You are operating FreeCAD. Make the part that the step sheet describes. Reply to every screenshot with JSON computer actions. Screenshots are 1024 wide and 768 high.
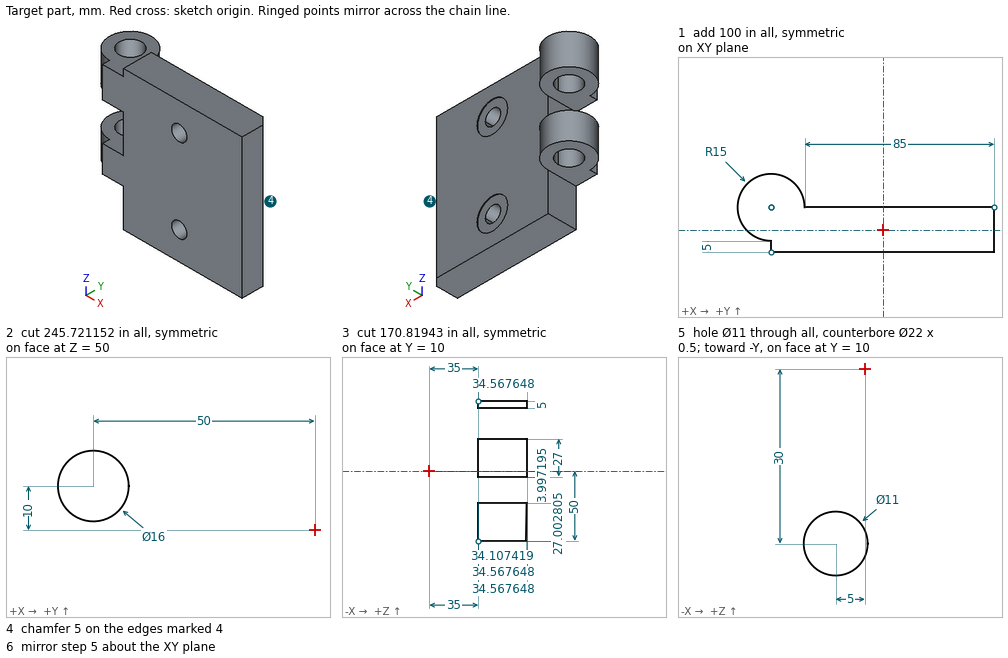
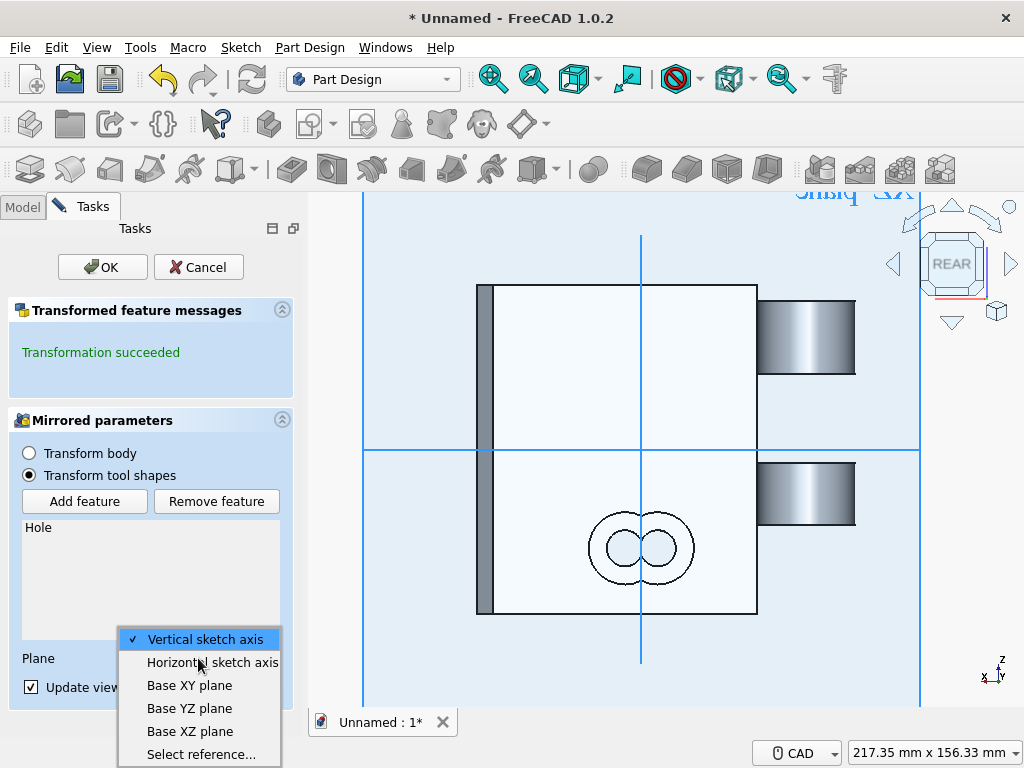
{"action": "left_click", "coordinate": [198, 686]}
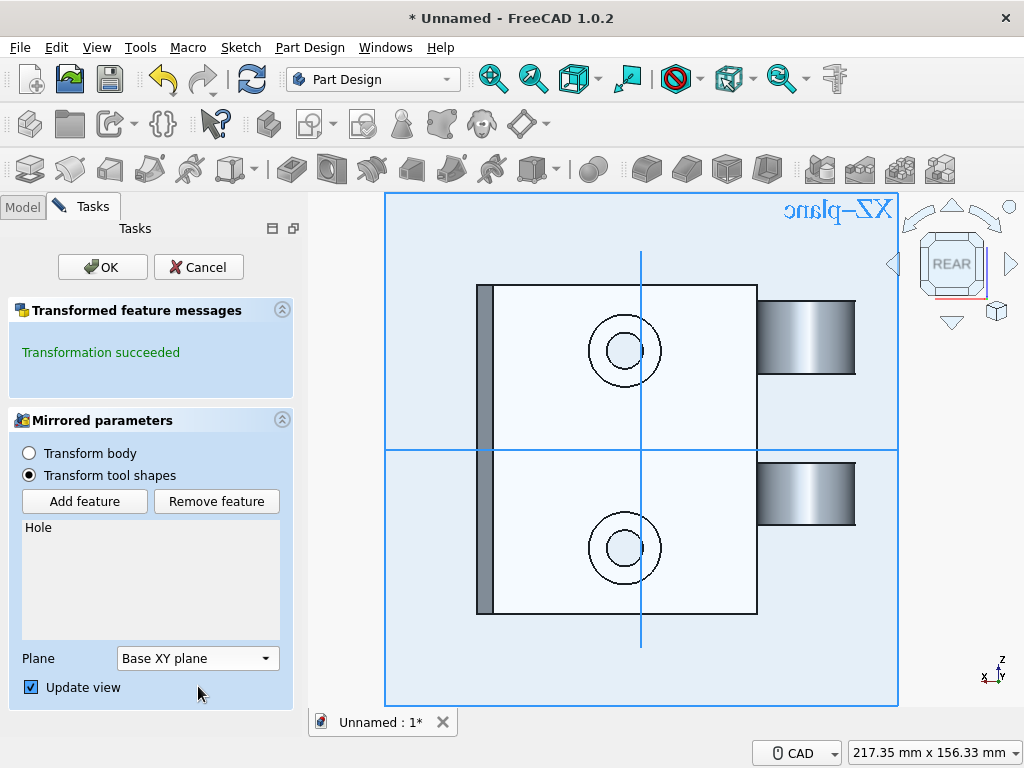
{"action": "left_click", "coordinate": [103, 267]}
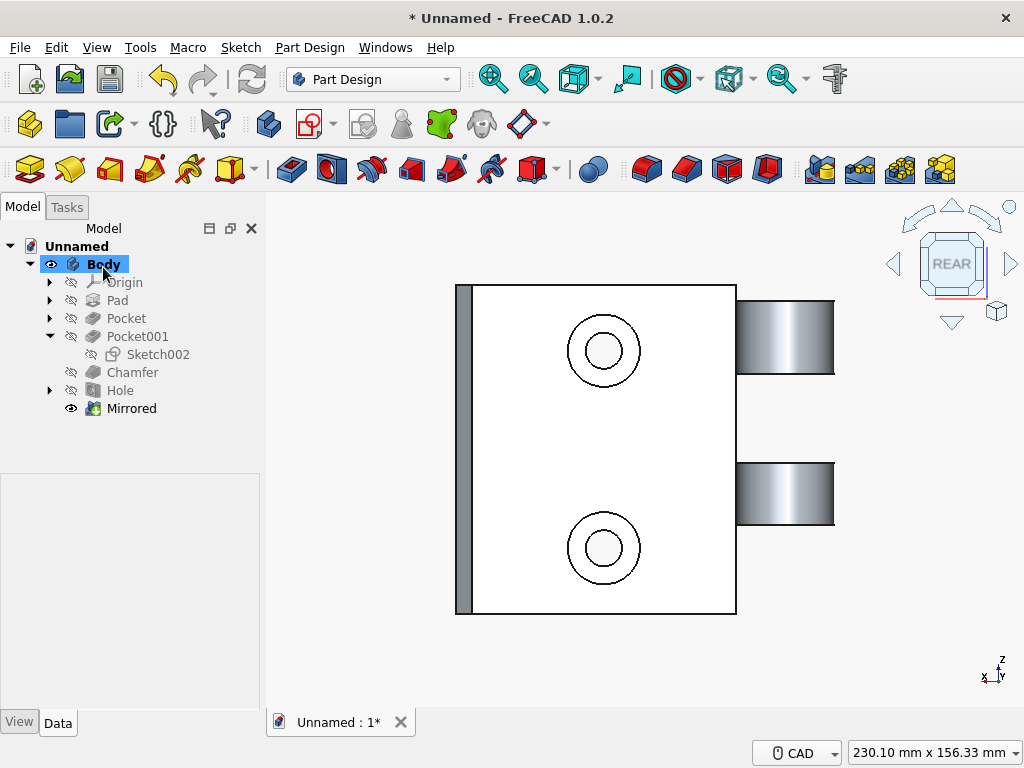
{"action": "key", "text": "0"}